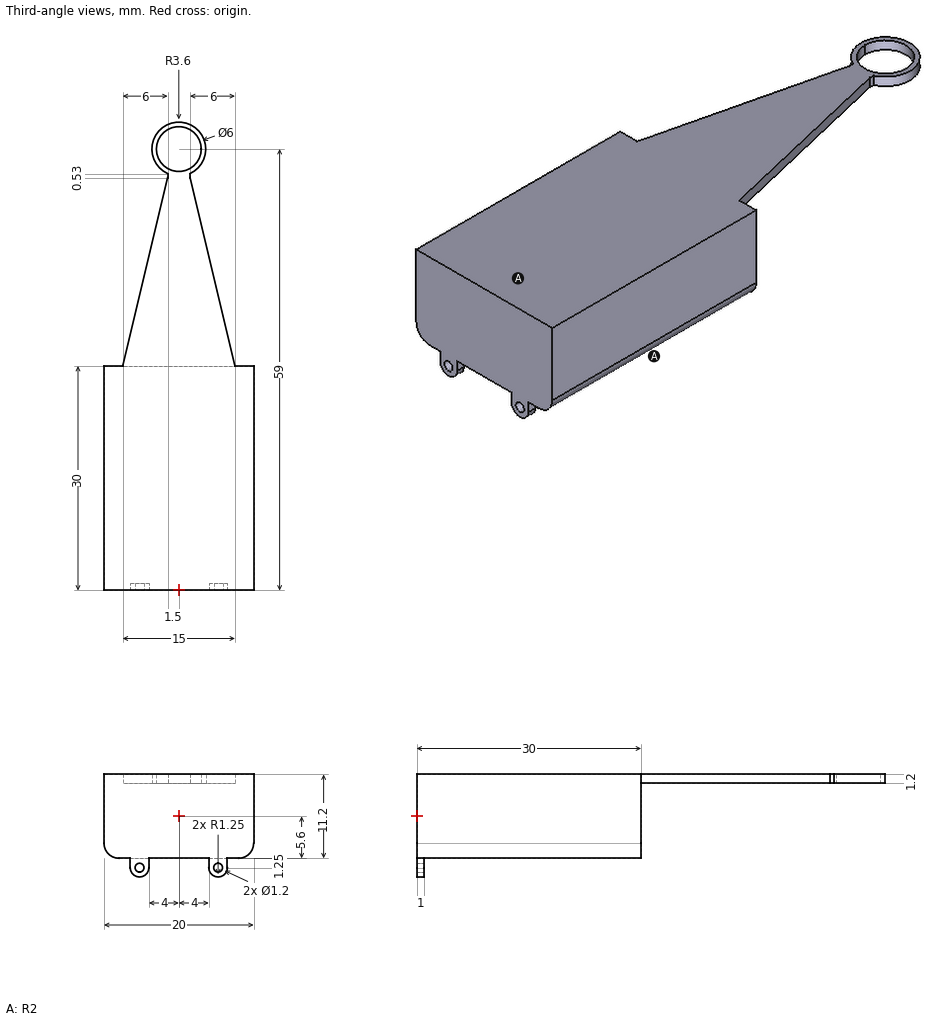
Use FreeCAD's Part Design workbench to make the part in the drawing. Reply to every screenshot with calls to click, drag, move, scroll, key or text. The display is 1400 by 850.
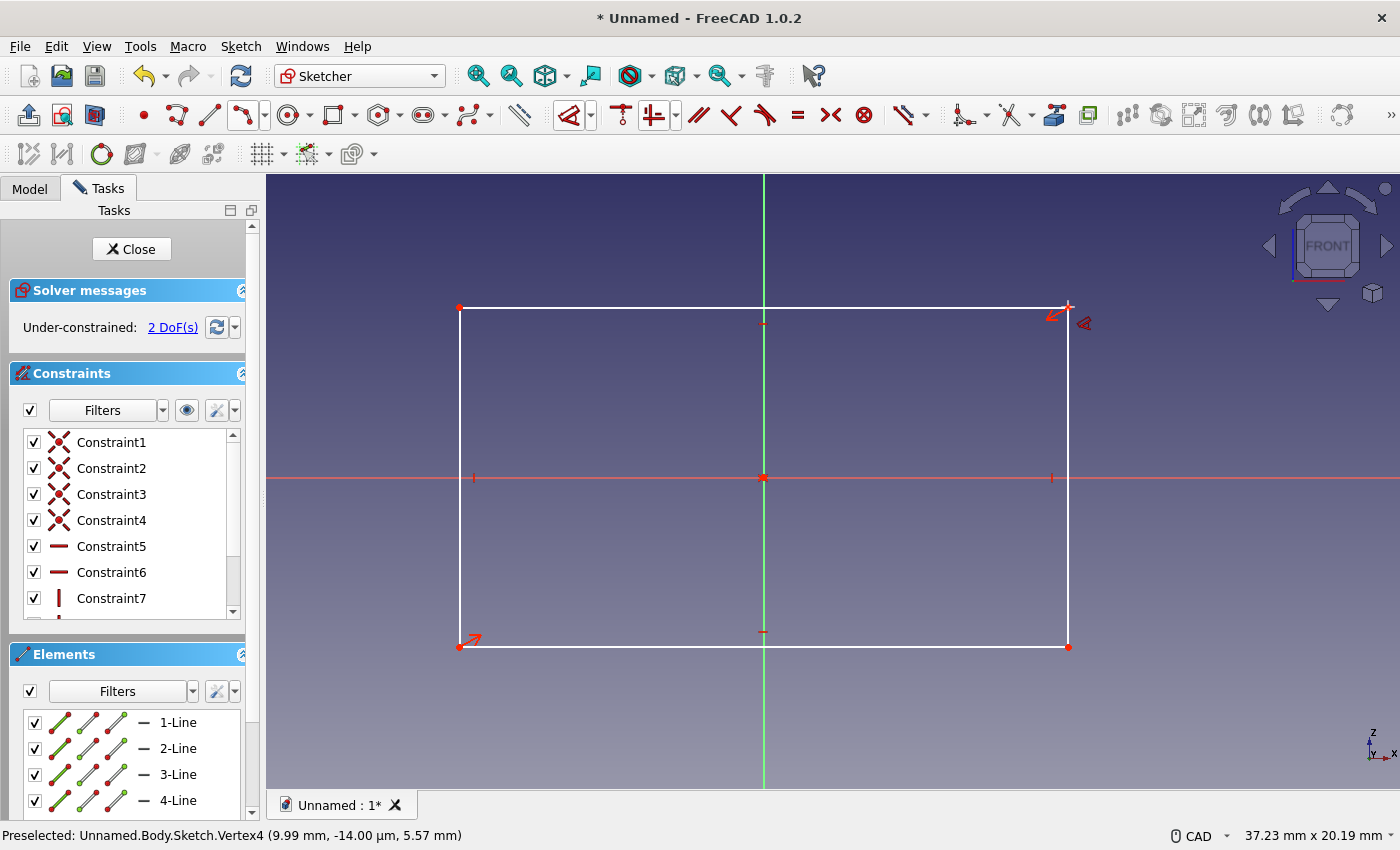
click(642, 647)
click(624, 681)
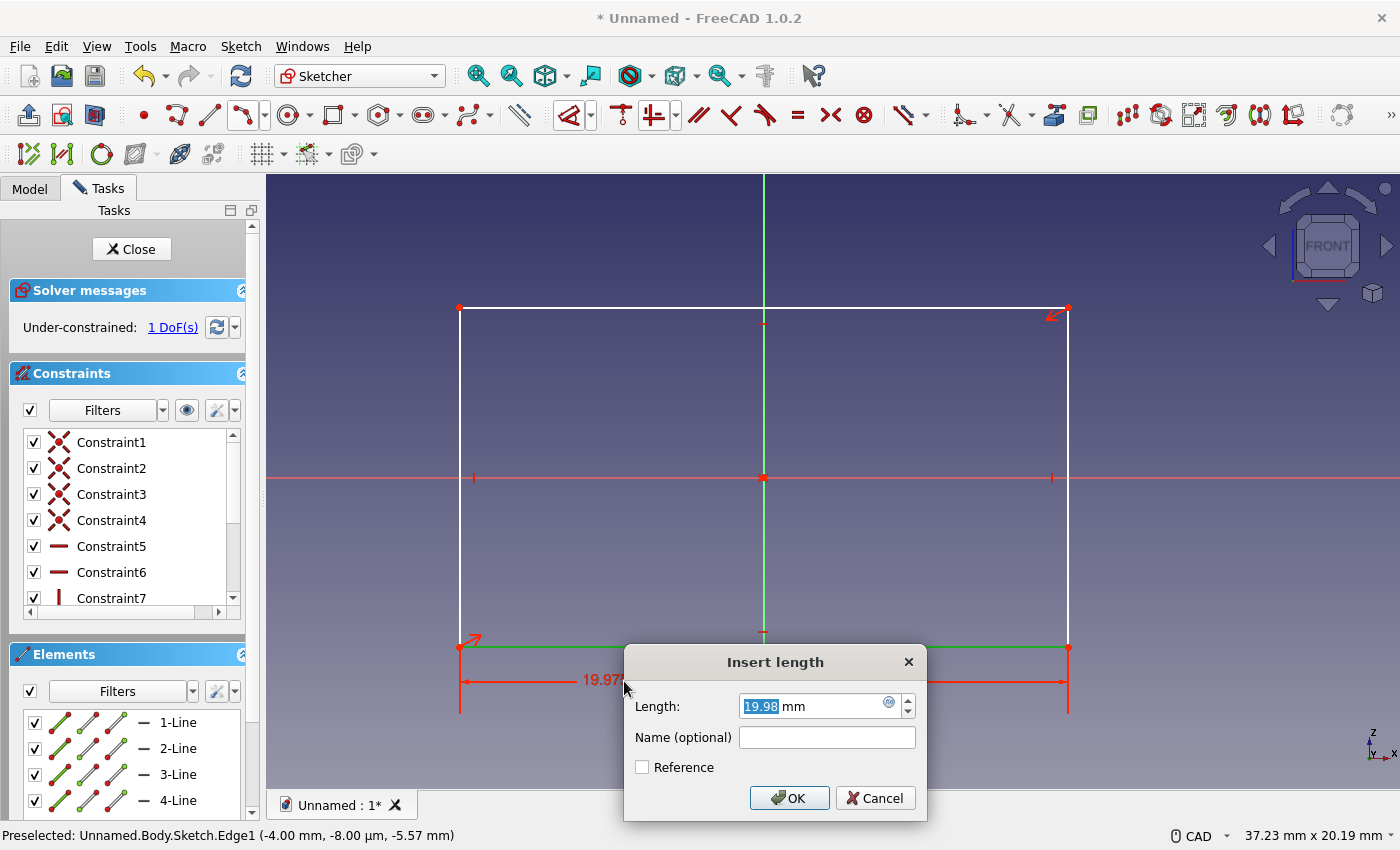
text(20)
key(Return)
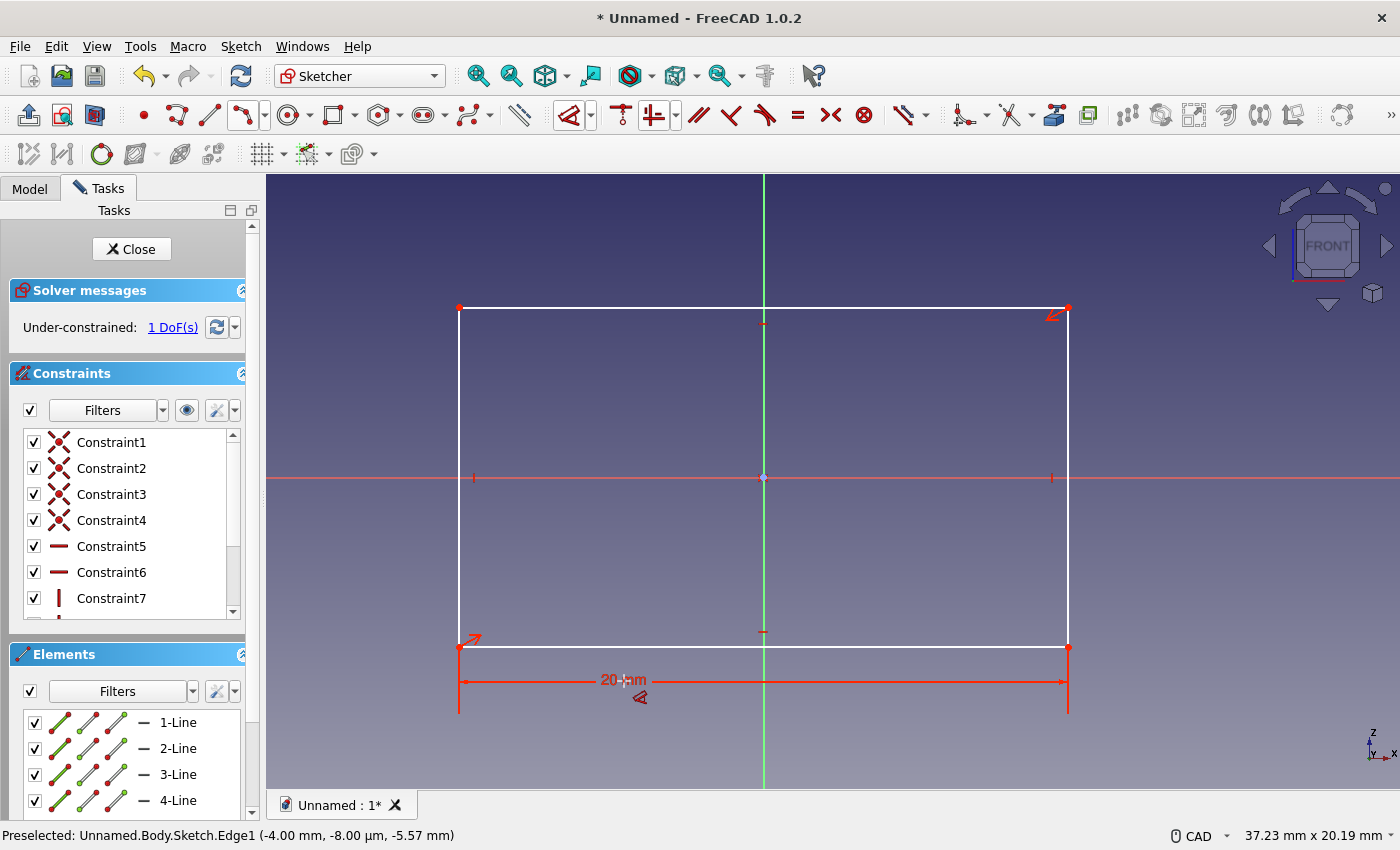
click(1068, 545)
click(1102, 400)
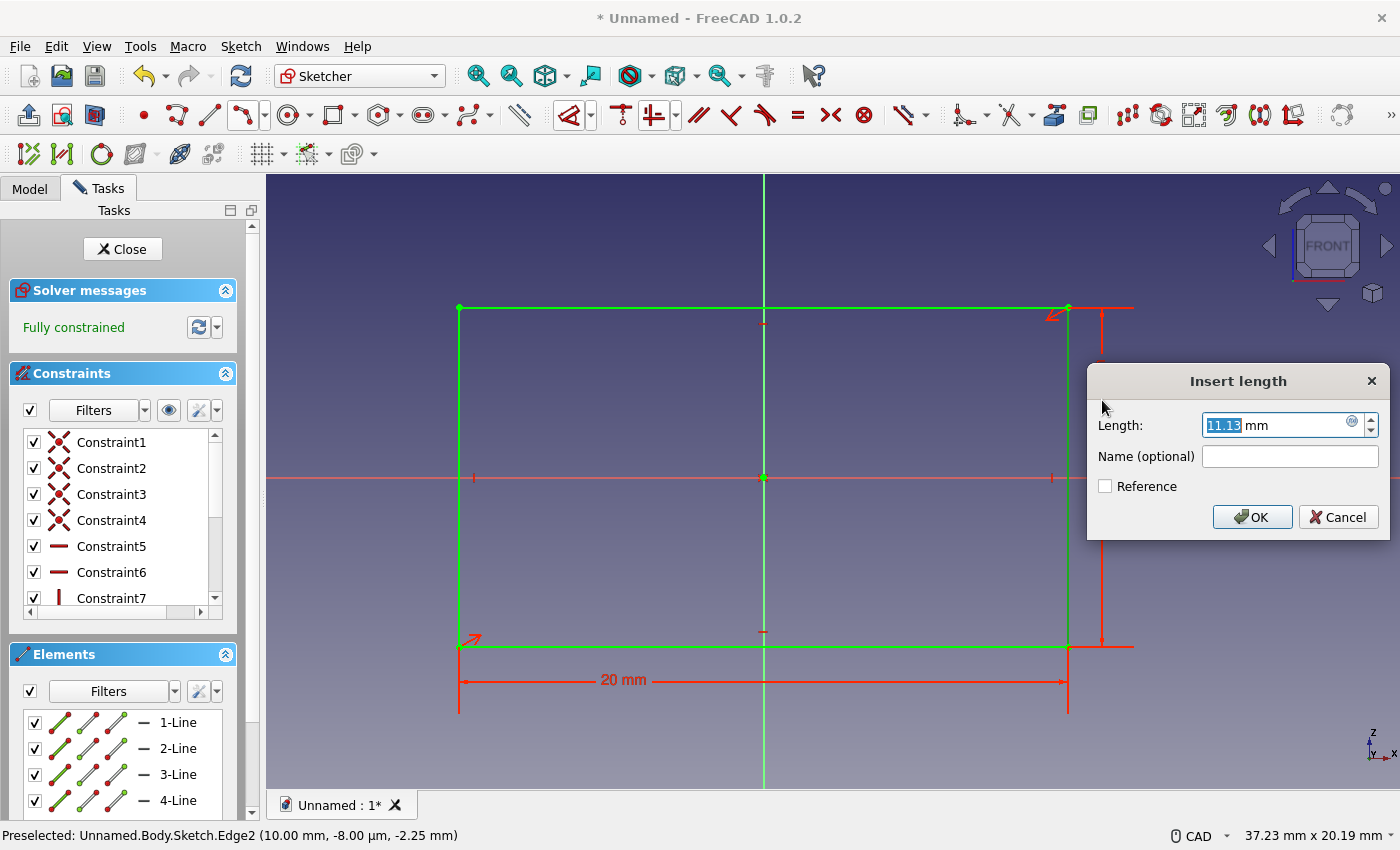
text(11.2)
key(Return)
key(Escape)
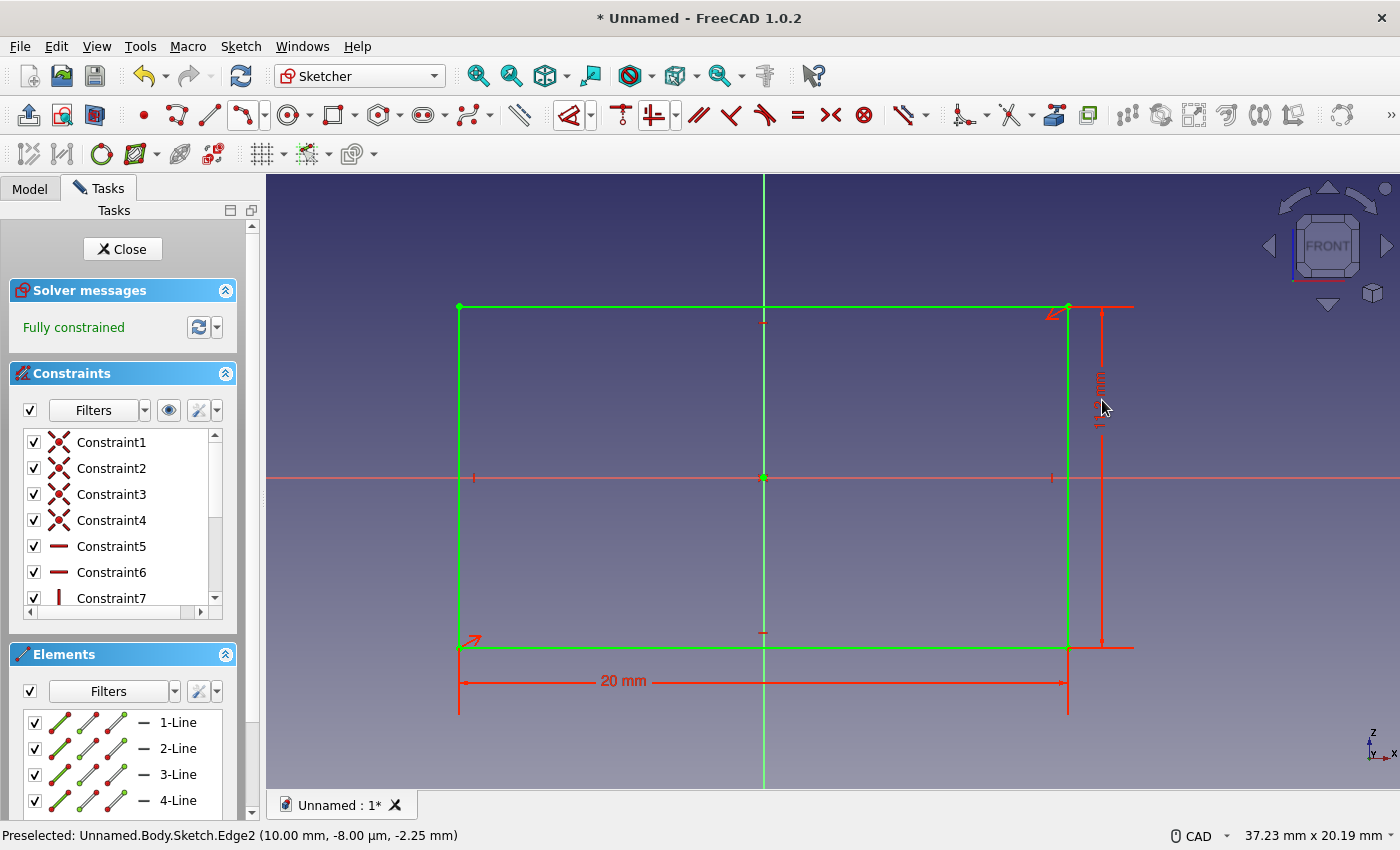
click(123, 249)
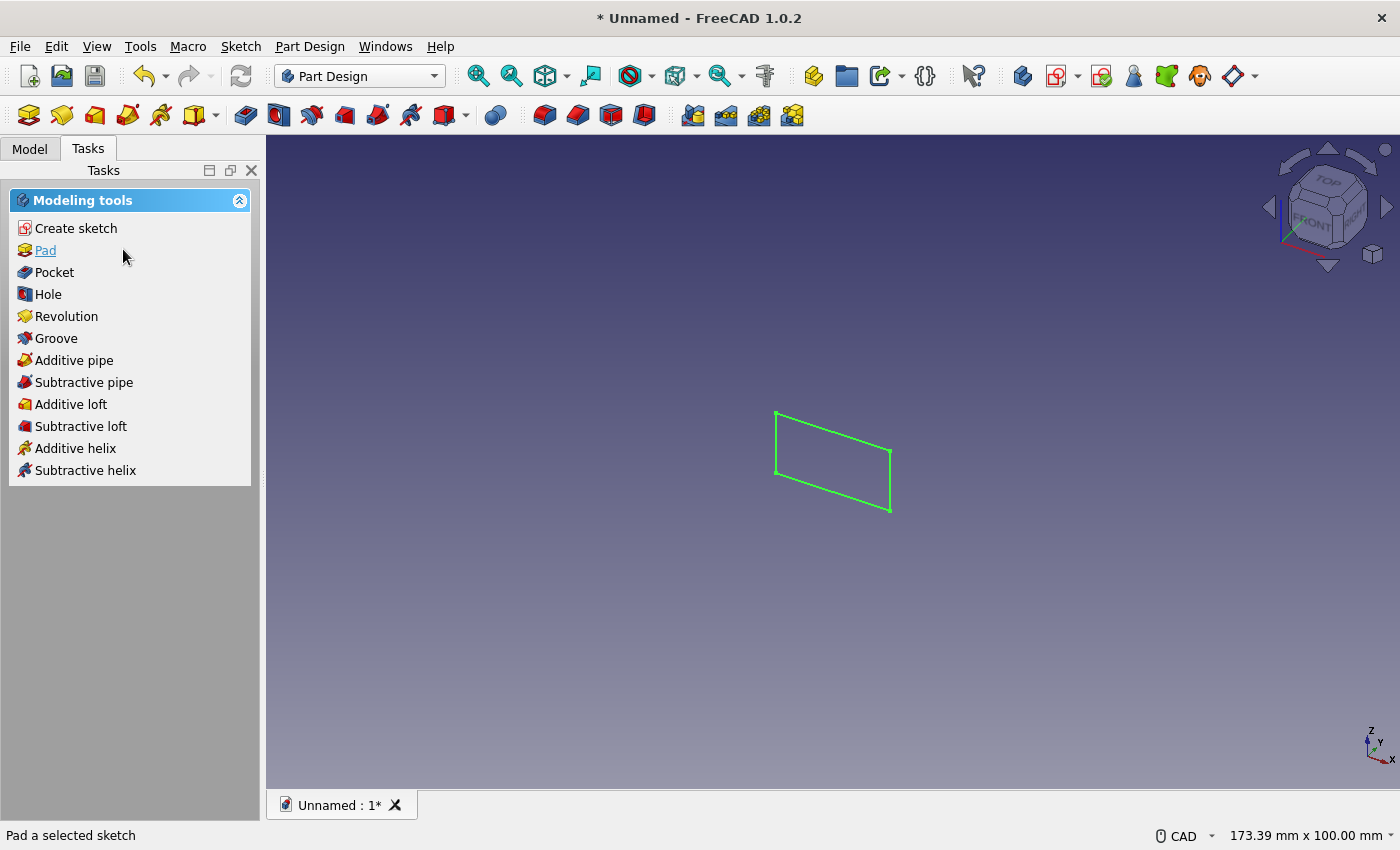
click(29, 116)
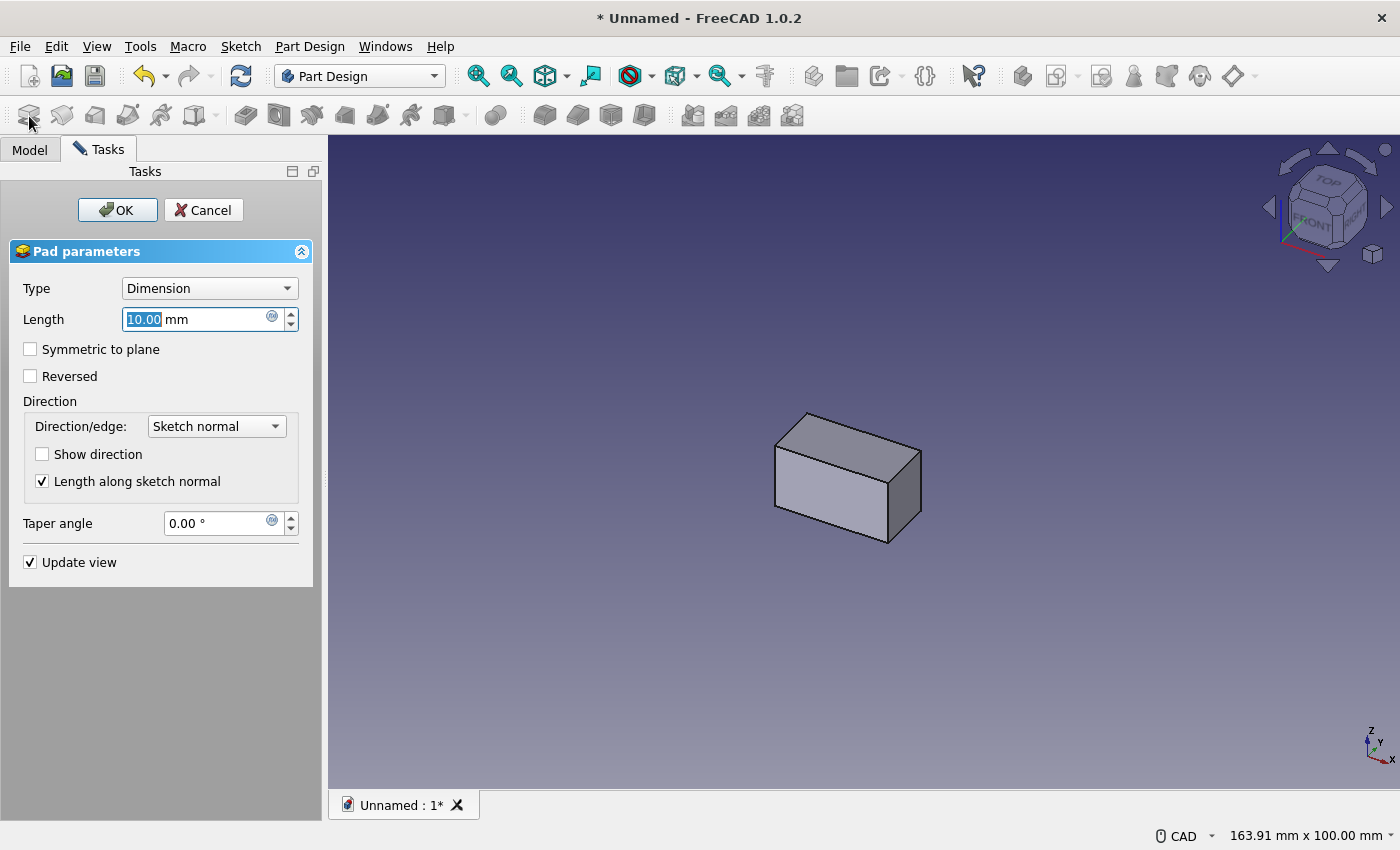
text(30)
key(Tab)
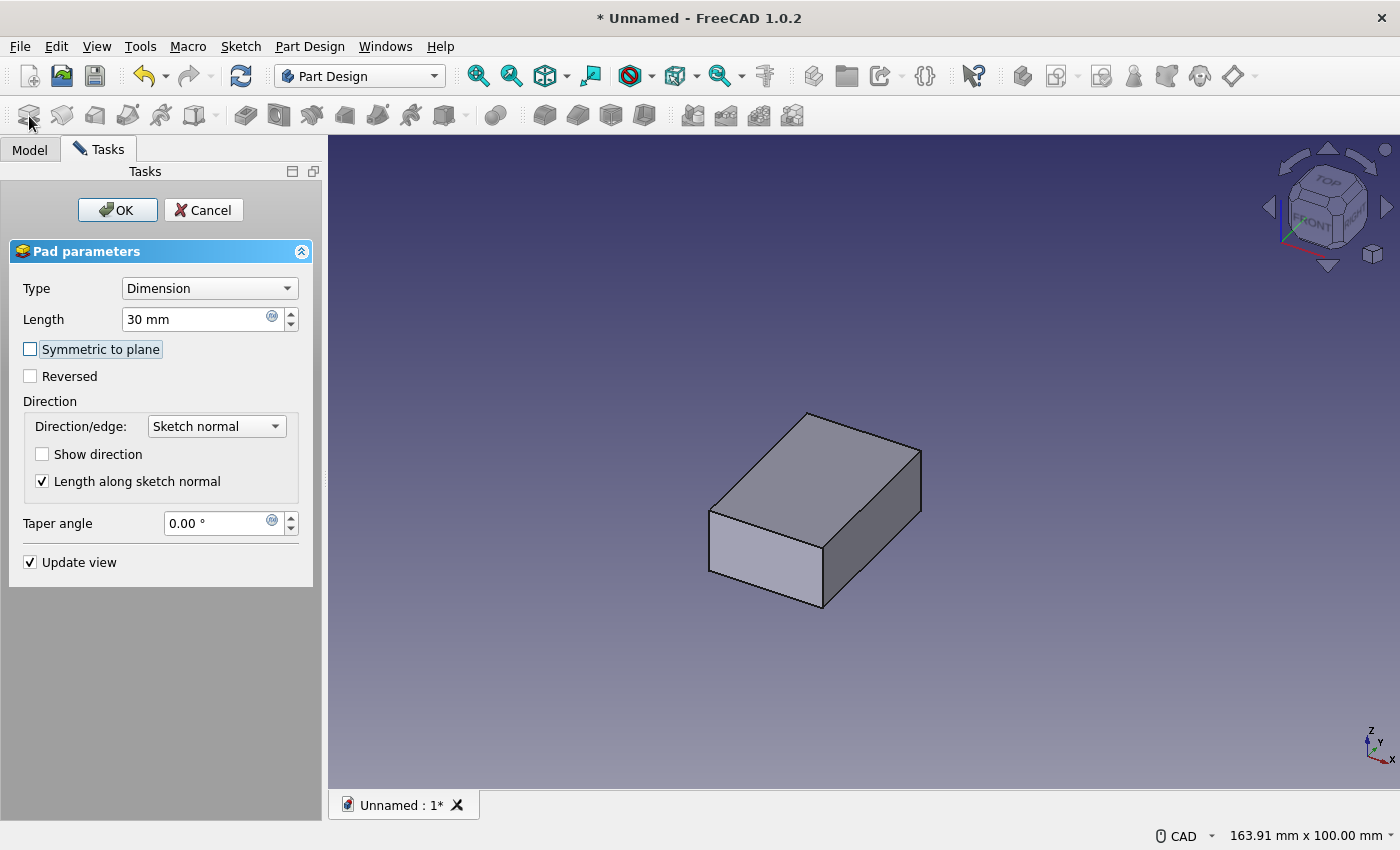
click(31, 376)